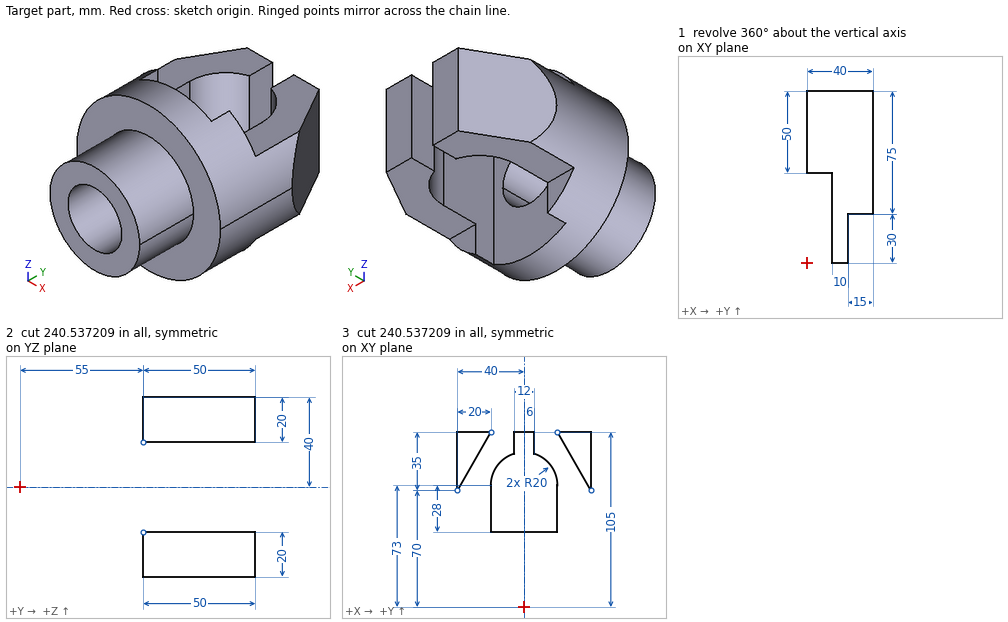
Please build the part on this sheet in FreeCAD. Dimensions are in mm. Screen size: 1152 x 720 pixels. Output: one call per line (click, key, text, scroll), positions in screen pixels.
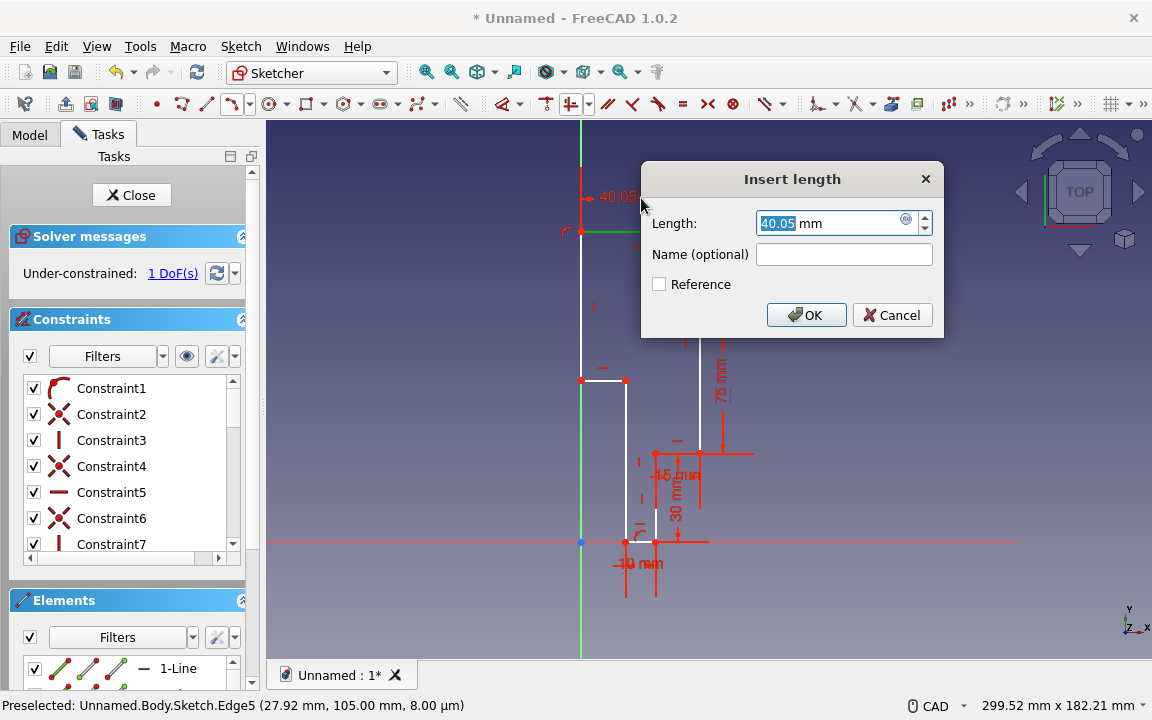
text(40)
key(Return)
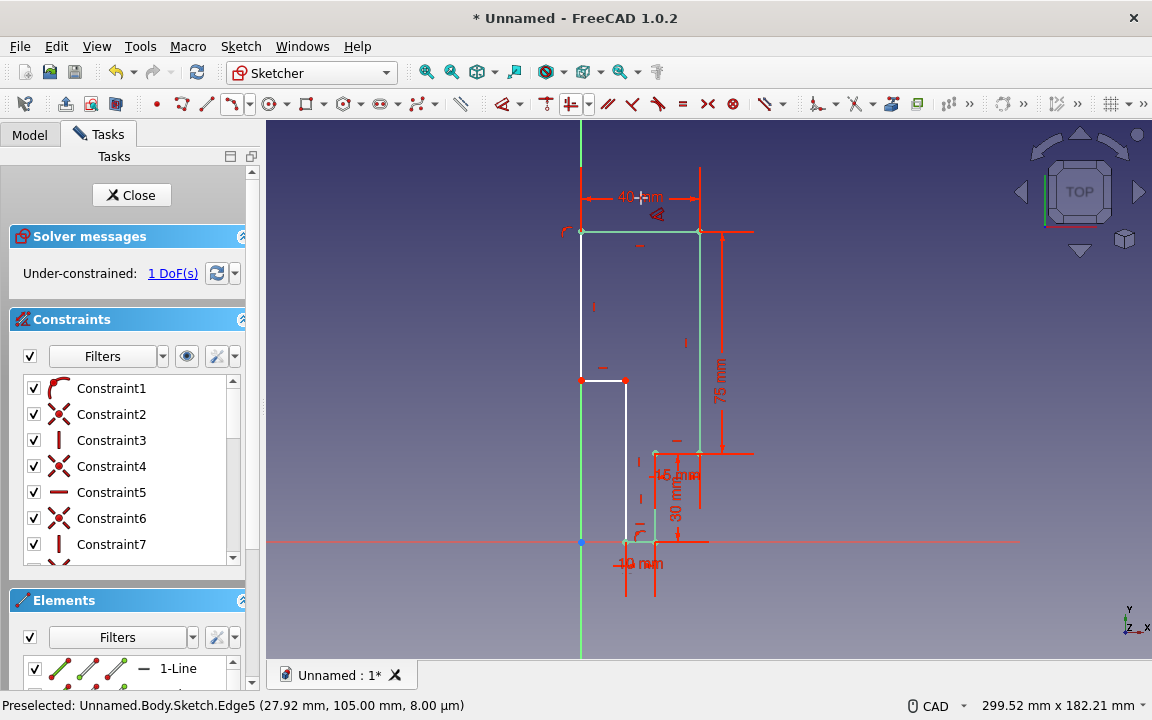
click(581, 277)
click(547, 306)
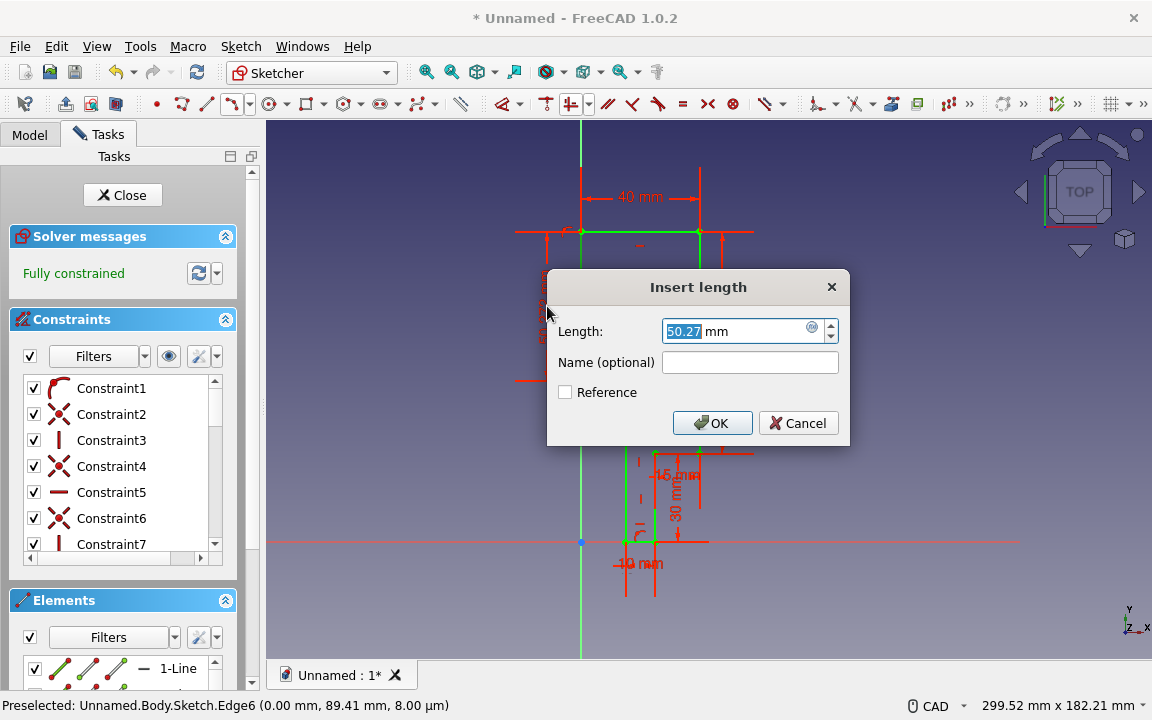
text(50)
key(Return)
key(Escape)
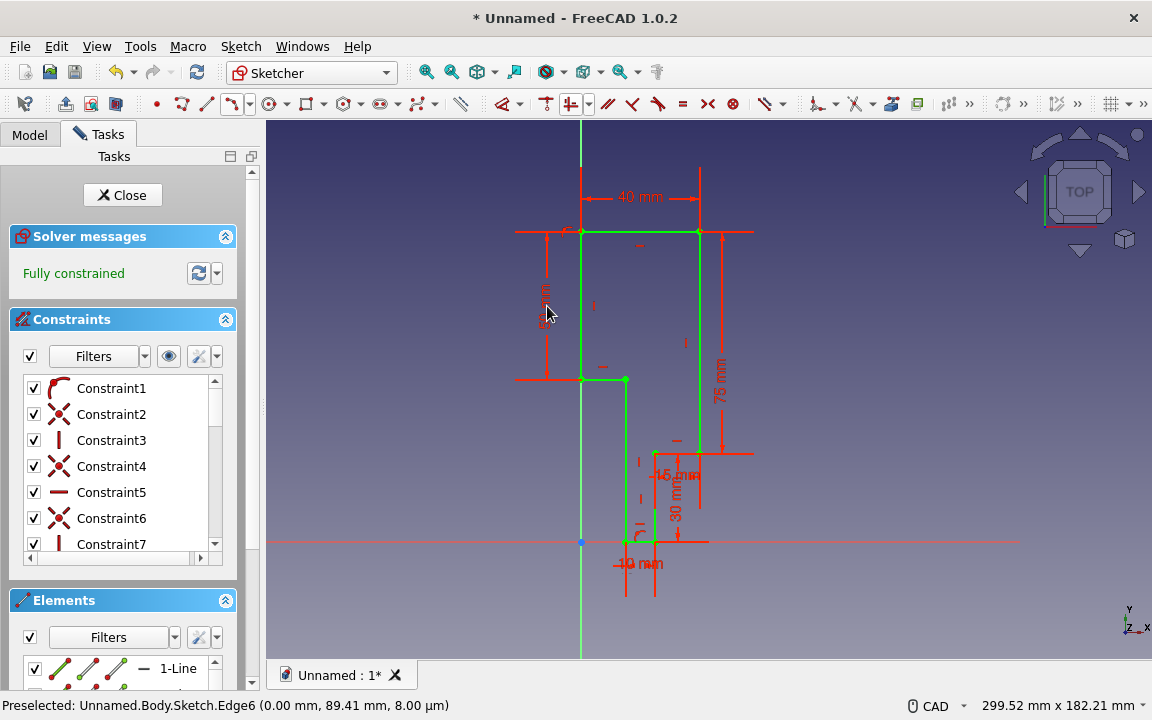
click(123, 195)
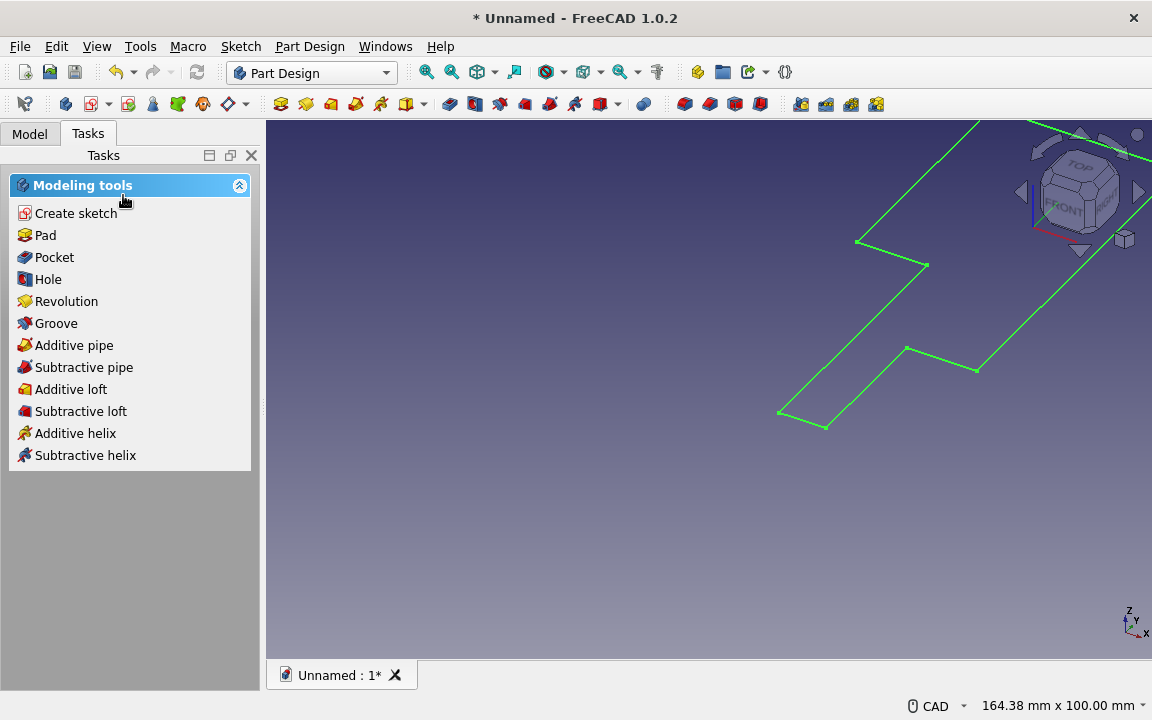
click(306, 104)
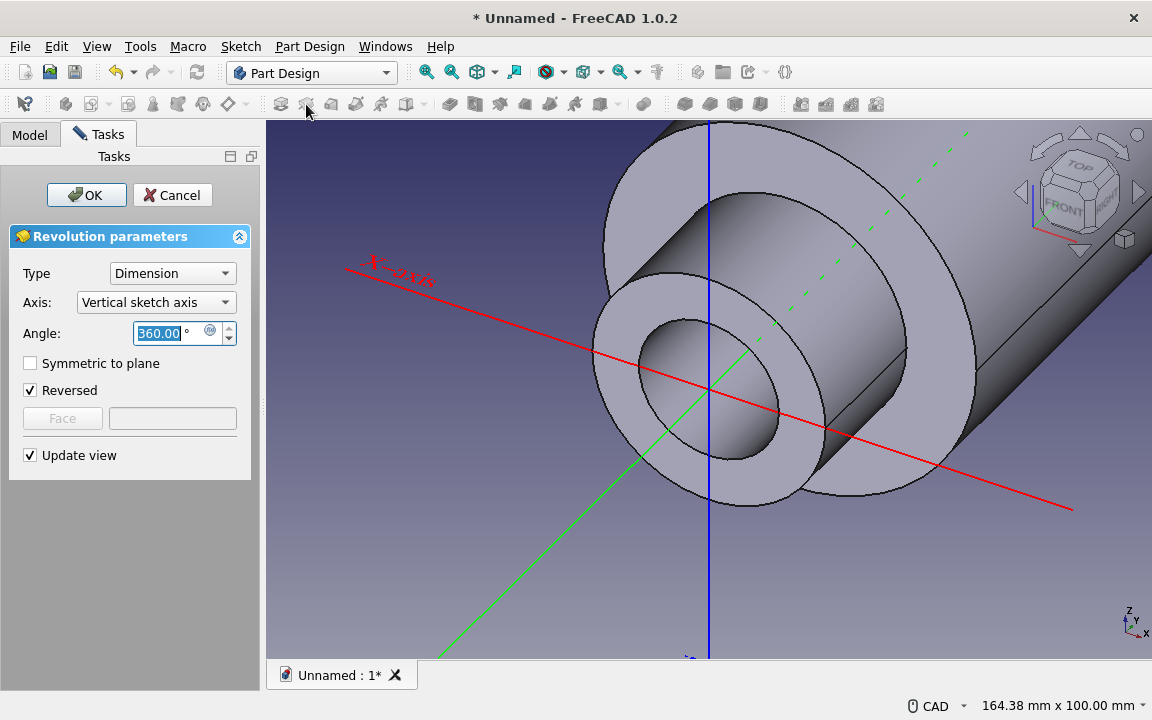
click(87, 195)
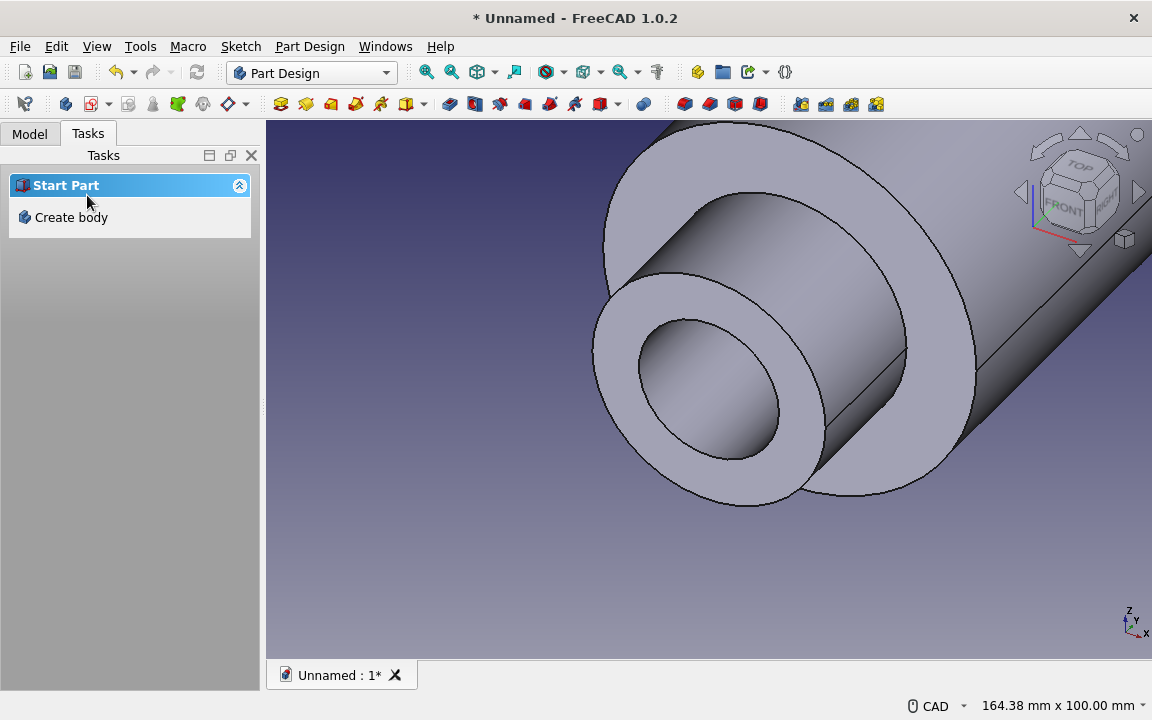
click(427, 72)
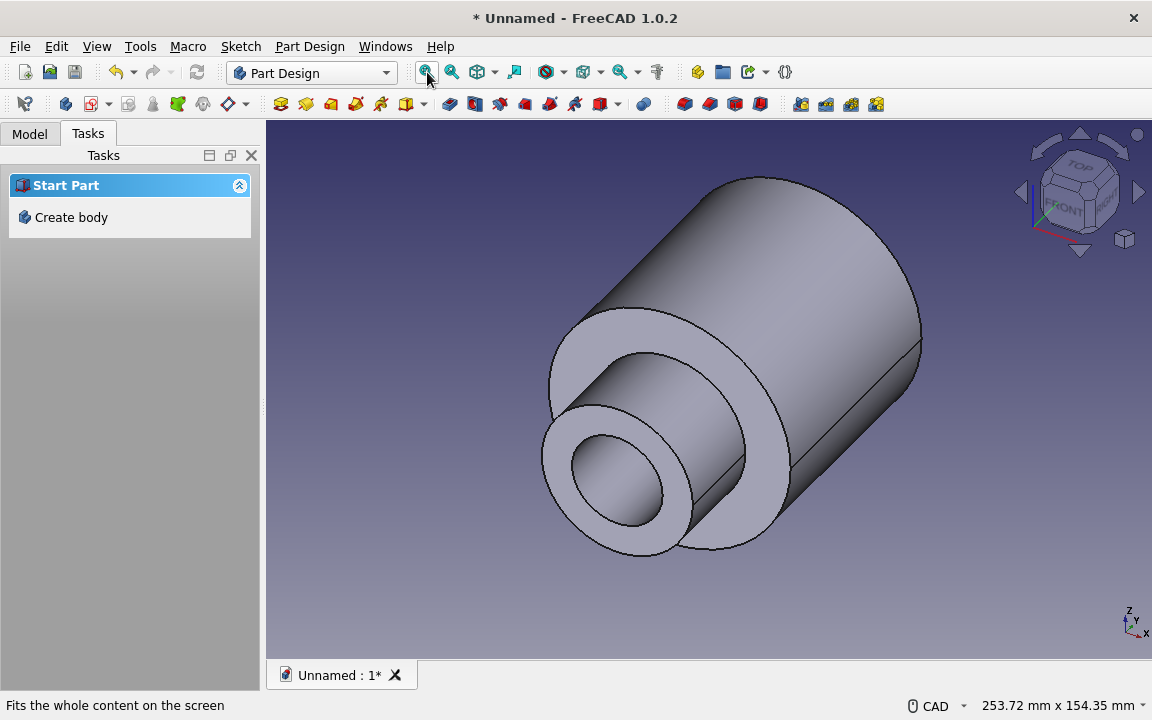
click(90, 104)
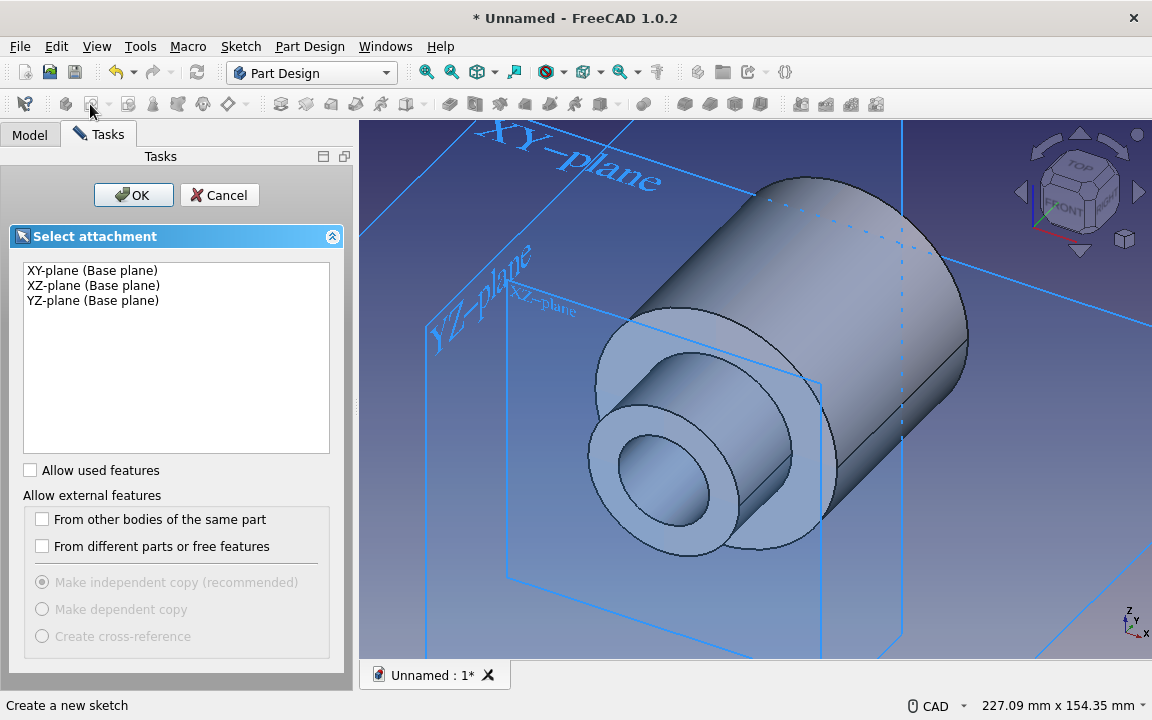
click(84, 300)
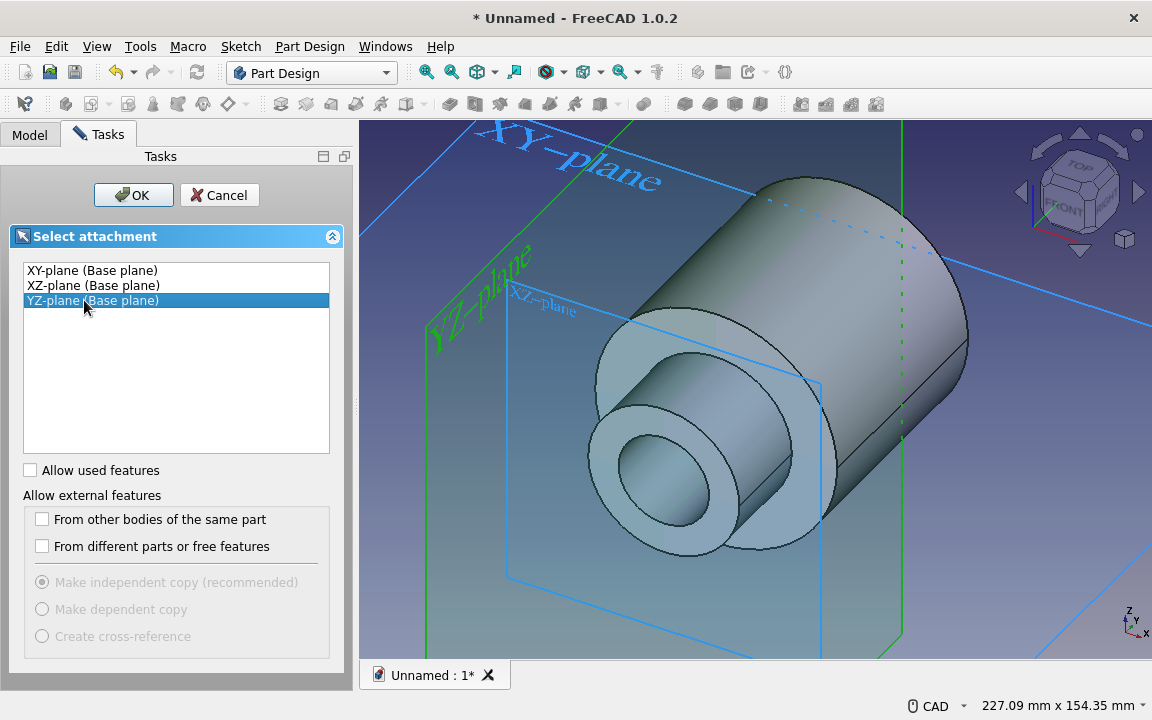
click(134, 195)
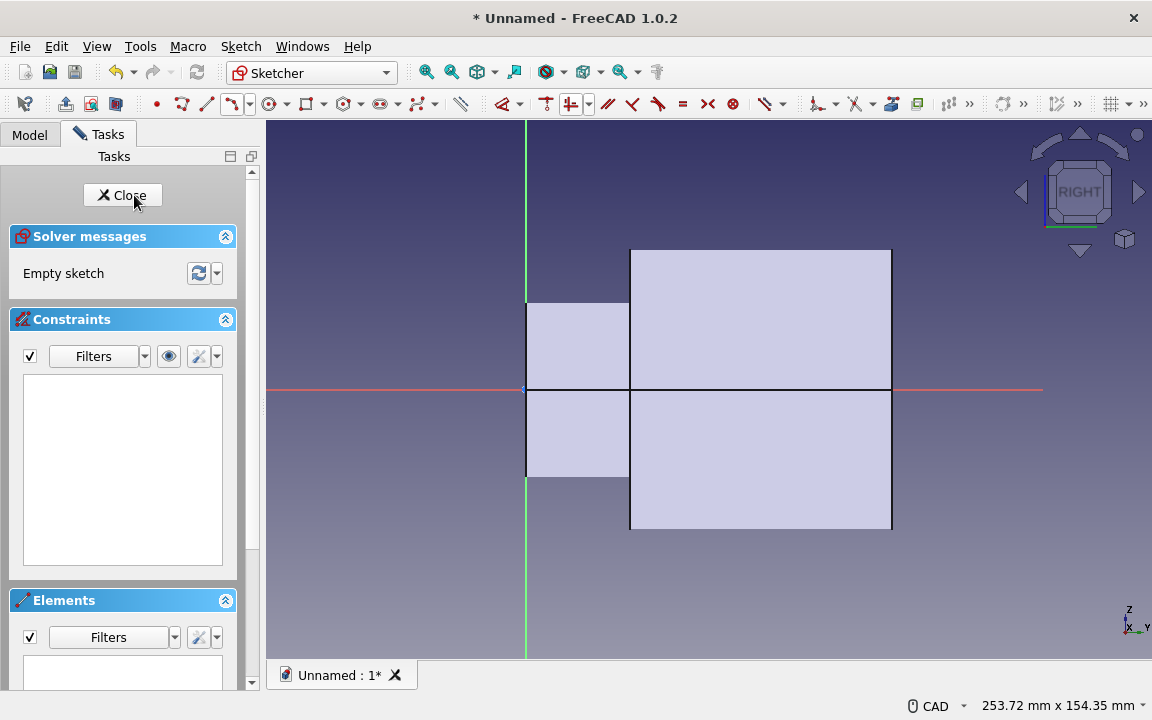
click(116, 104)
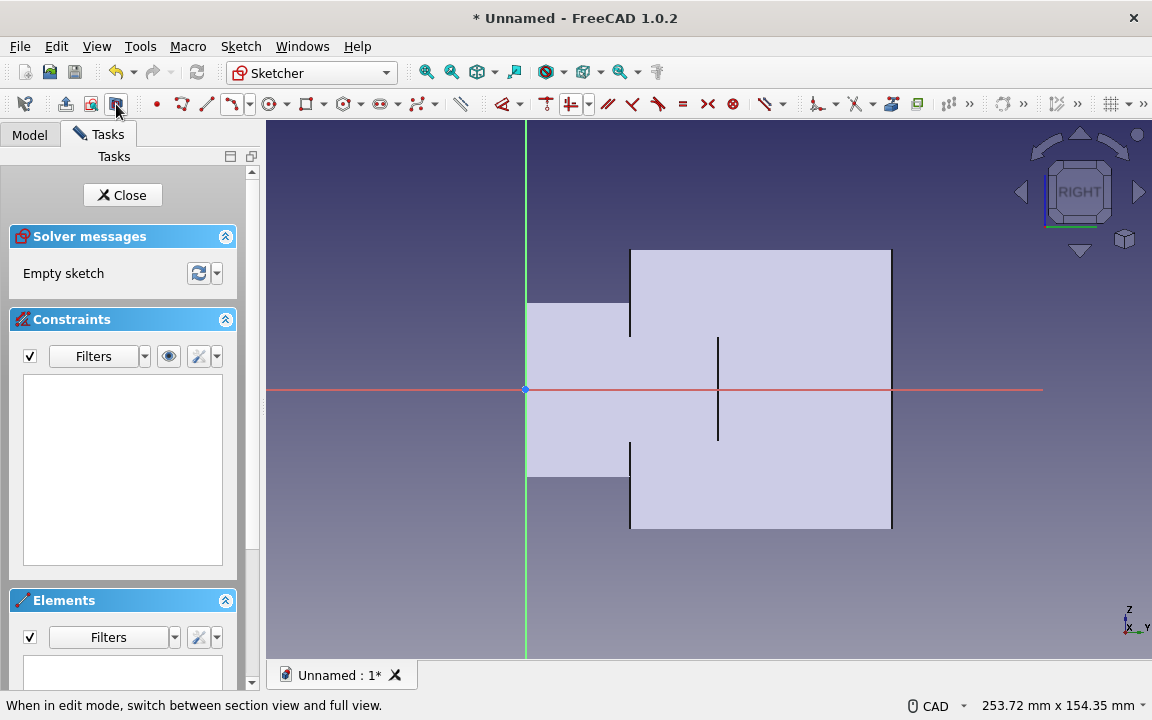
click(306, 104)